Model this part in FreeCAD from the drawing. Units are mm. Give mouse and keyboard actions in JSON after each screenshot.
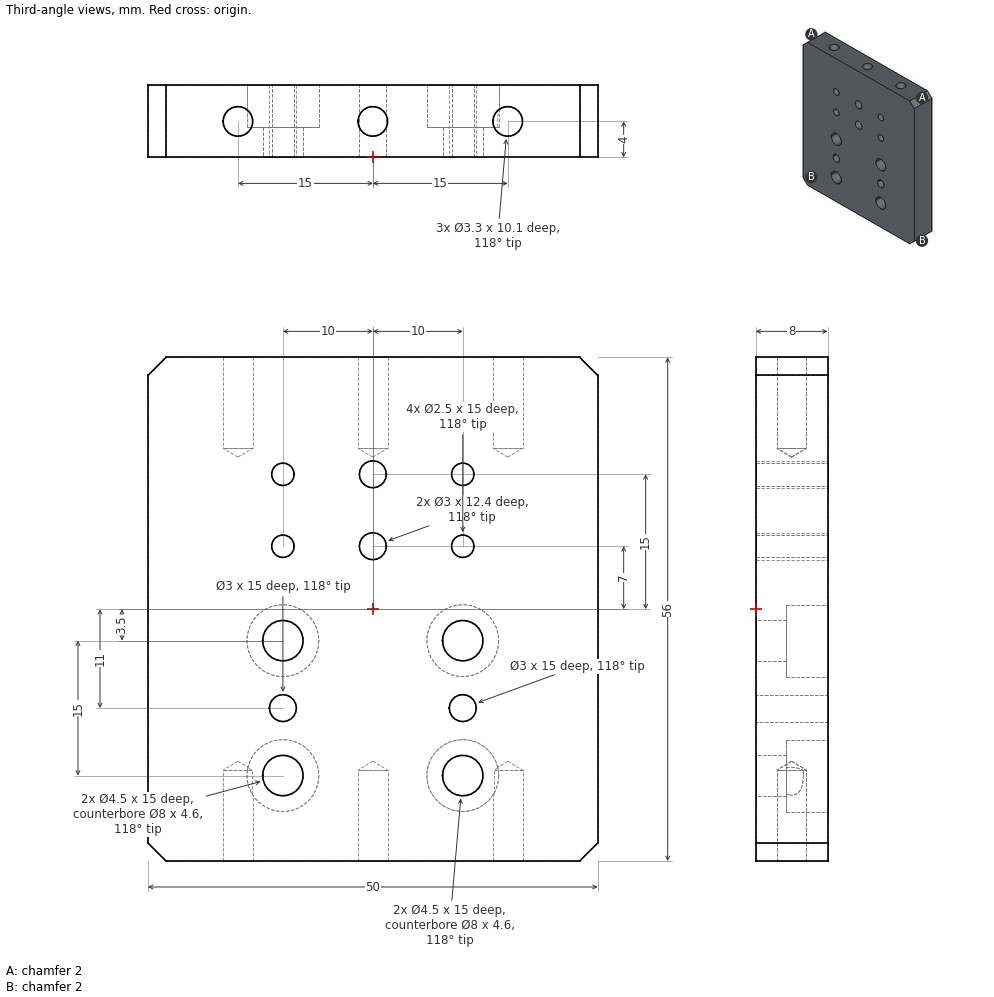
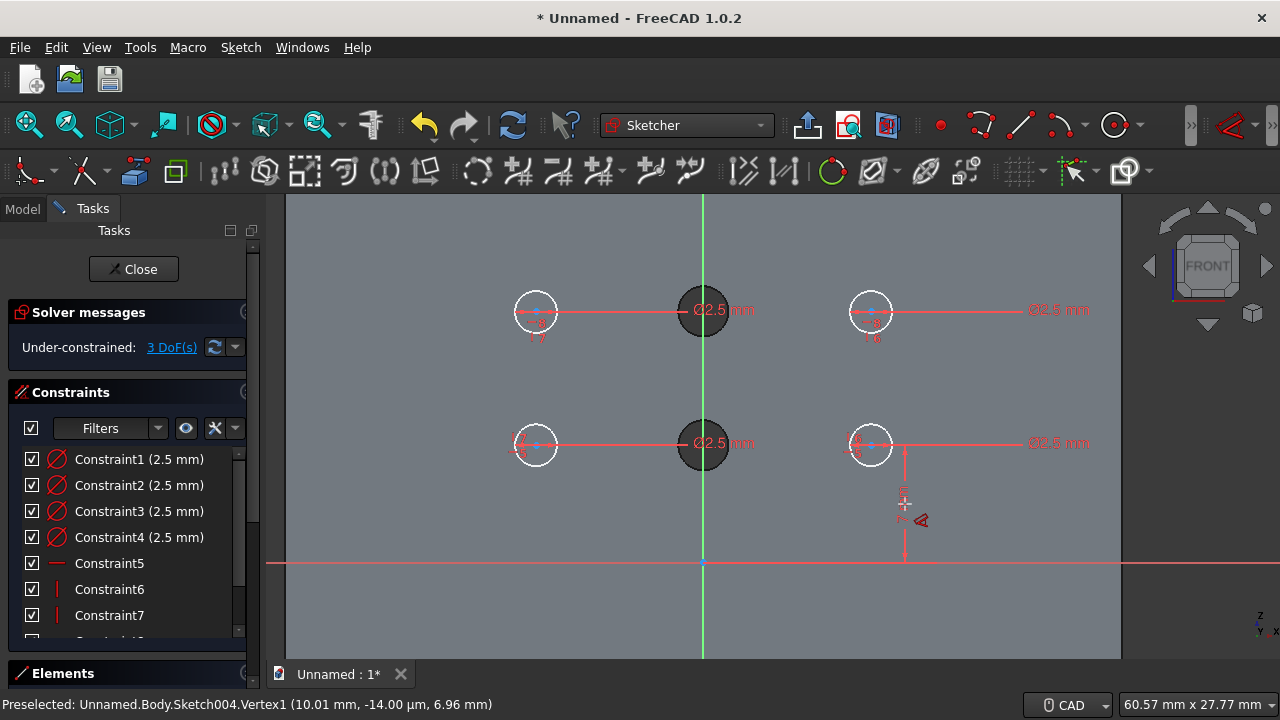
{"action": "left_click", "coordinate": [871, 445]}
{"action": "left_click", "coordinate": [787, 597]}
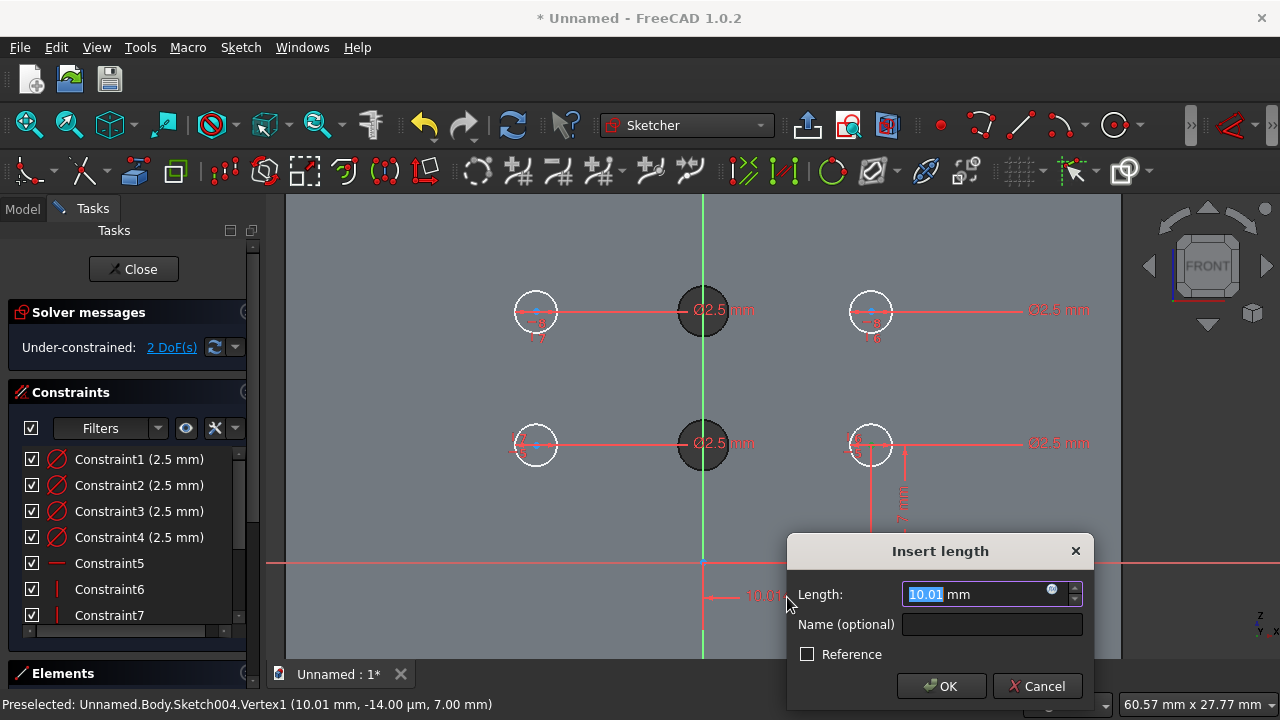
{"action": "type", "text": "10"}
{"action": "key", "text": "Return"}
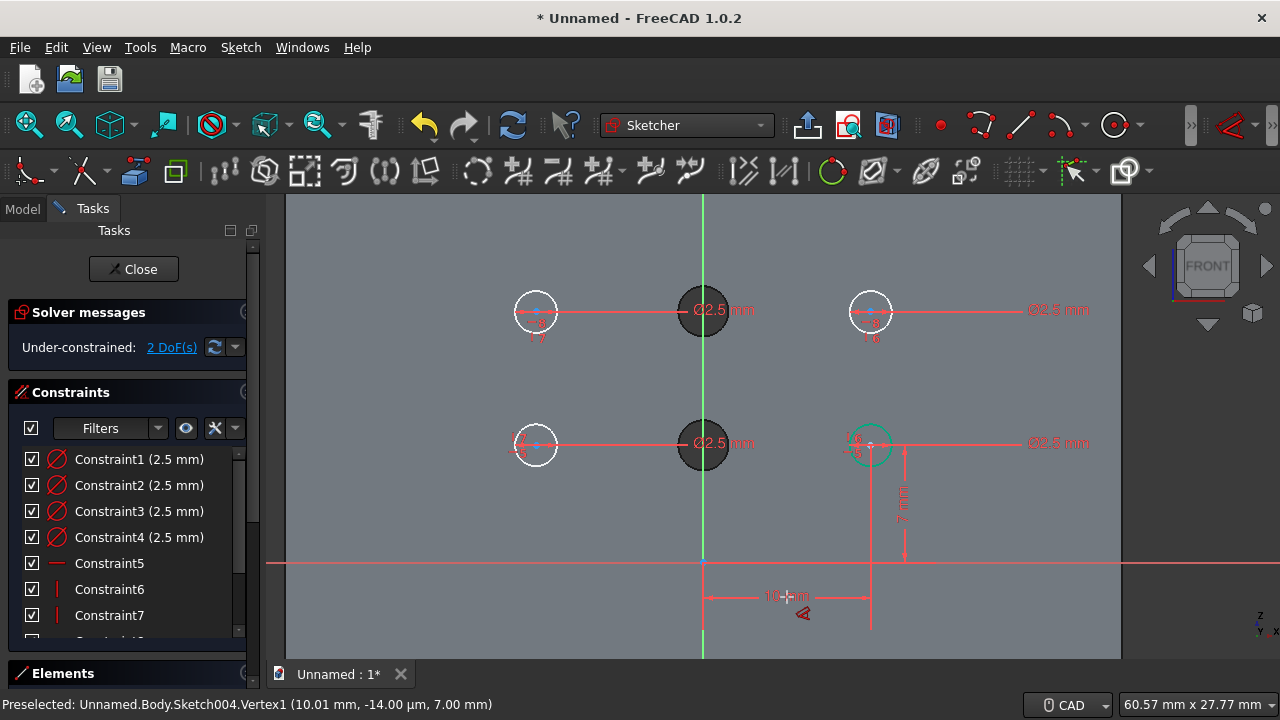
{"action": "left_click", "coordinate": [536, 445]}
{"action": "left_click", "coordinate": [620, 597]}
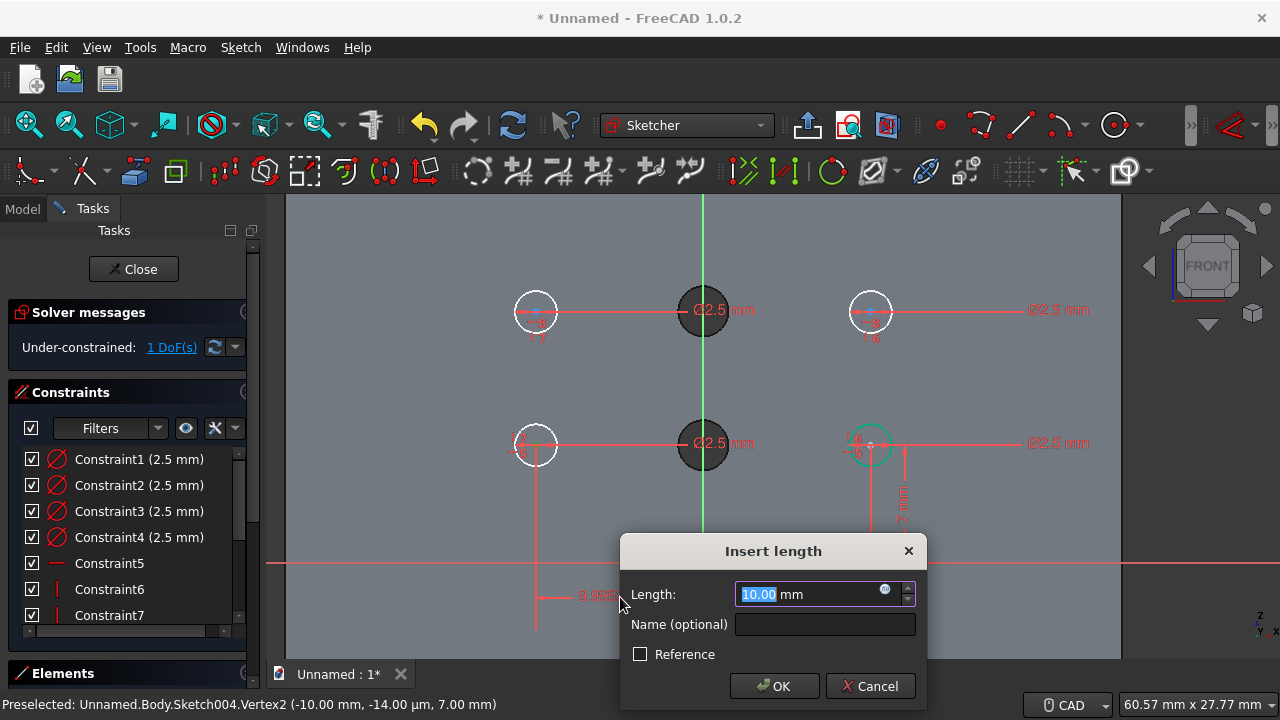
{"action": "type", "text": "10"}
{"action": "key", "text": "Return"}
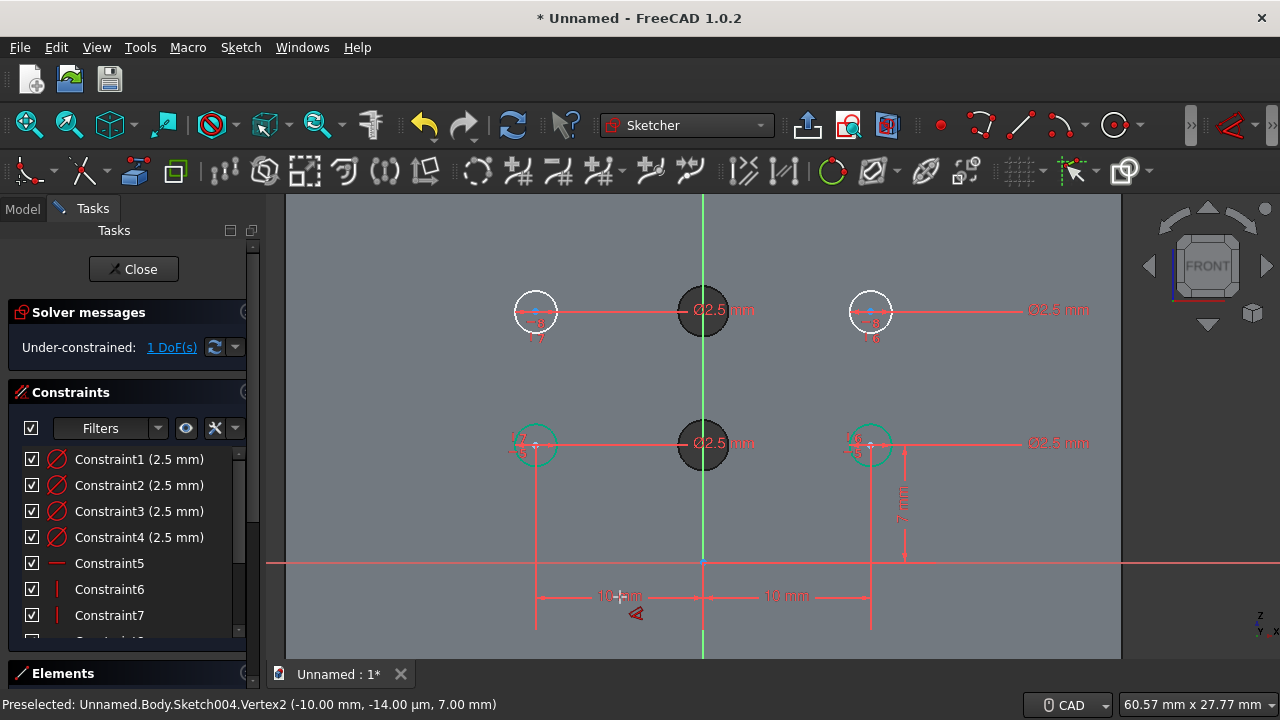
{"action": "left_click", "coordinate": [871, 312]}
{"action": "left_click", "coordinate": [905, 437]}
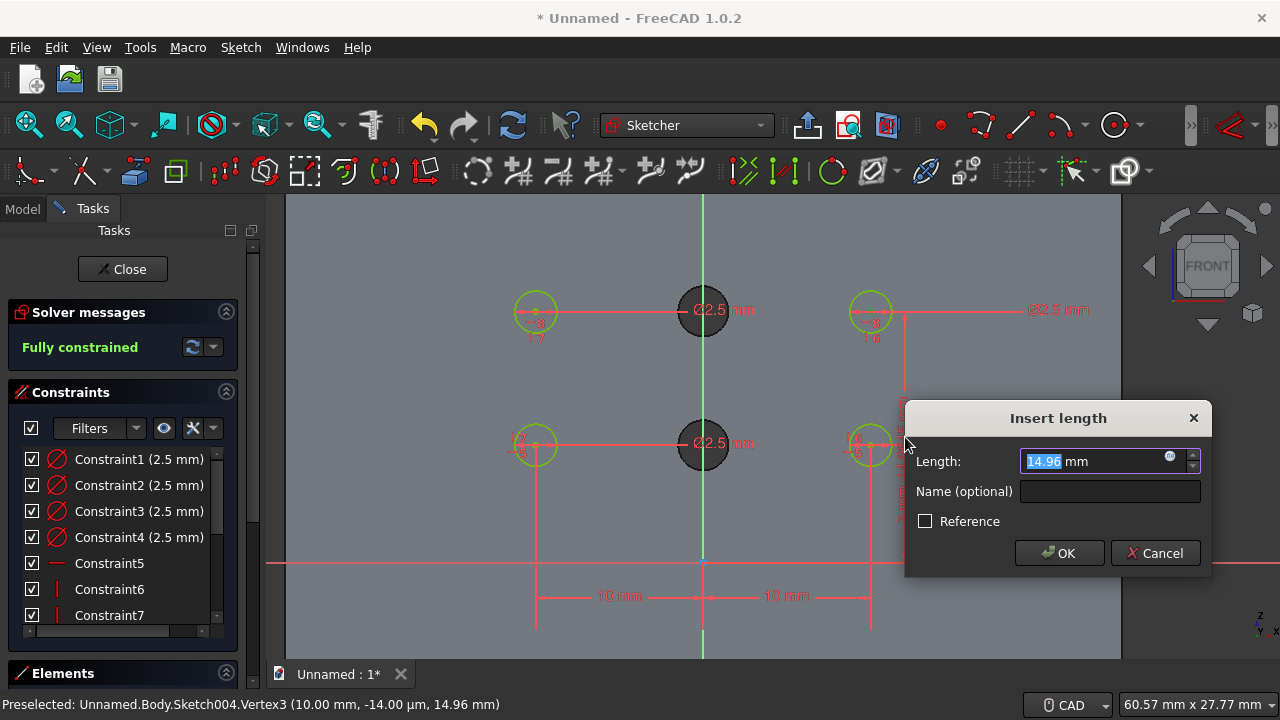
{"action": "type", "text": "15"}
{"action": "key", "text": "Return"}
{"action": "key", "text": "Escape"}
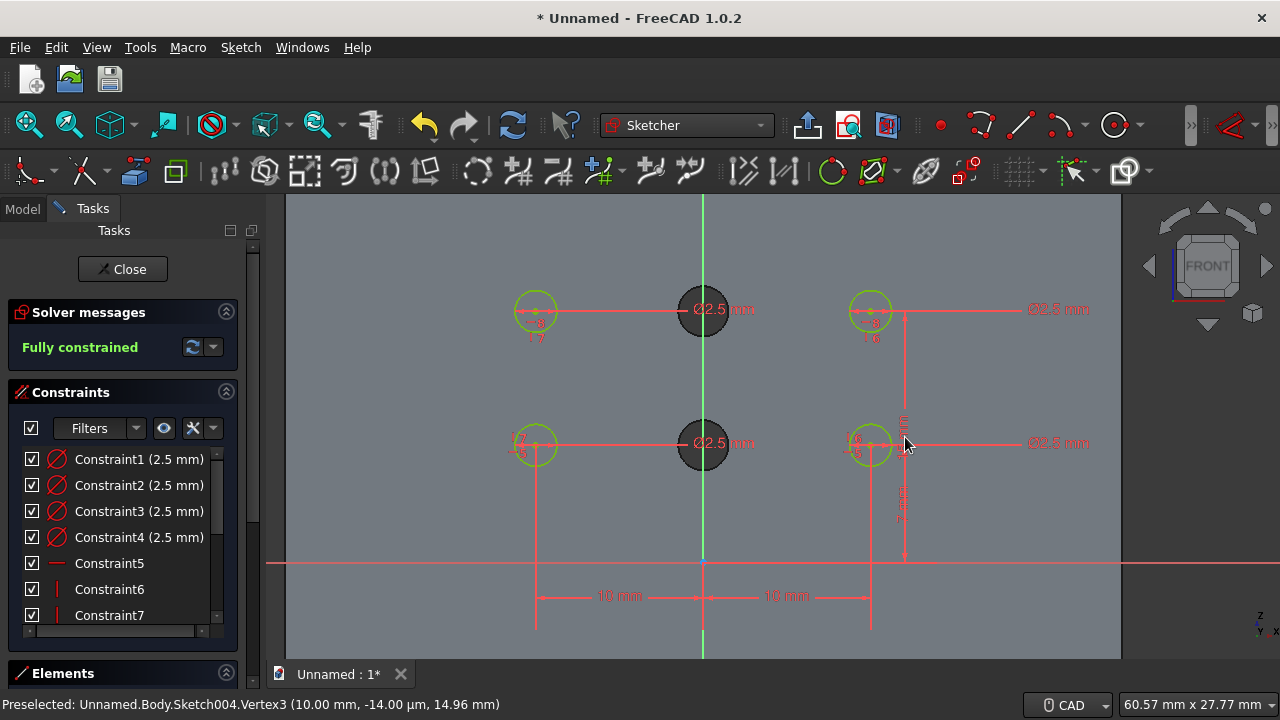
{"action": "left_click", "coordinate": [123, 269]}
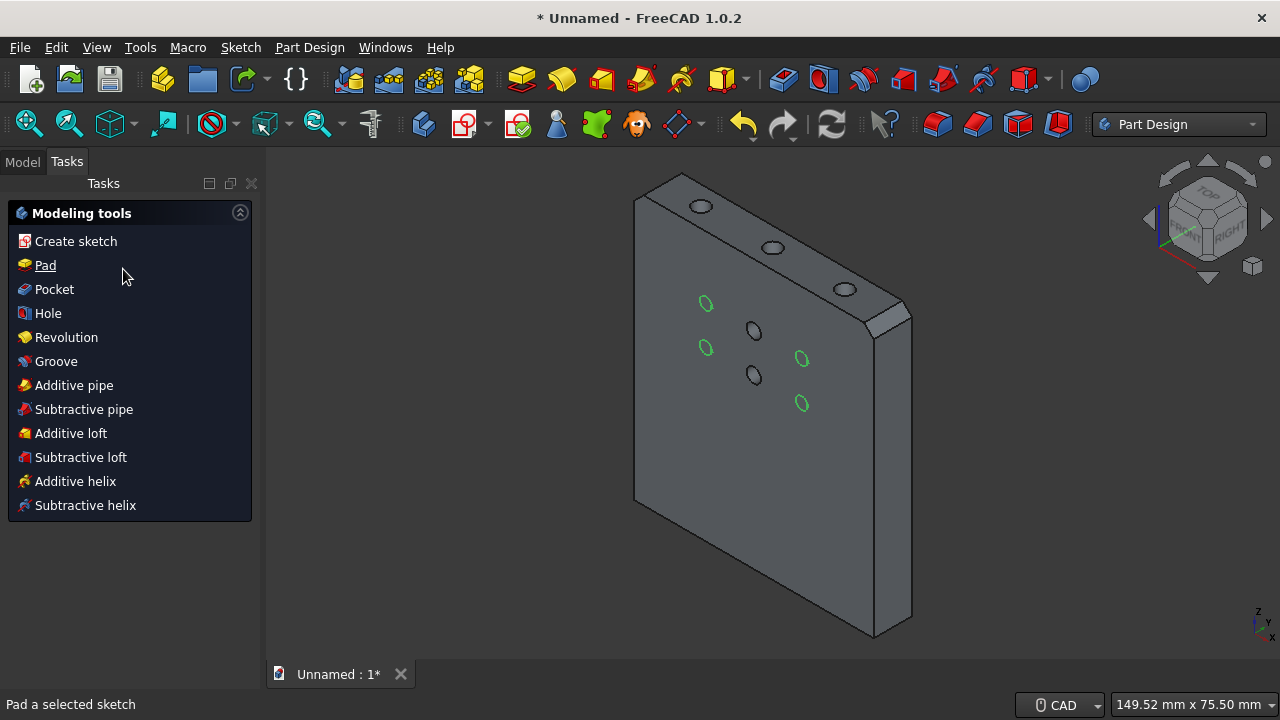
{"action": "left_click", "coordinate": [824, 80]}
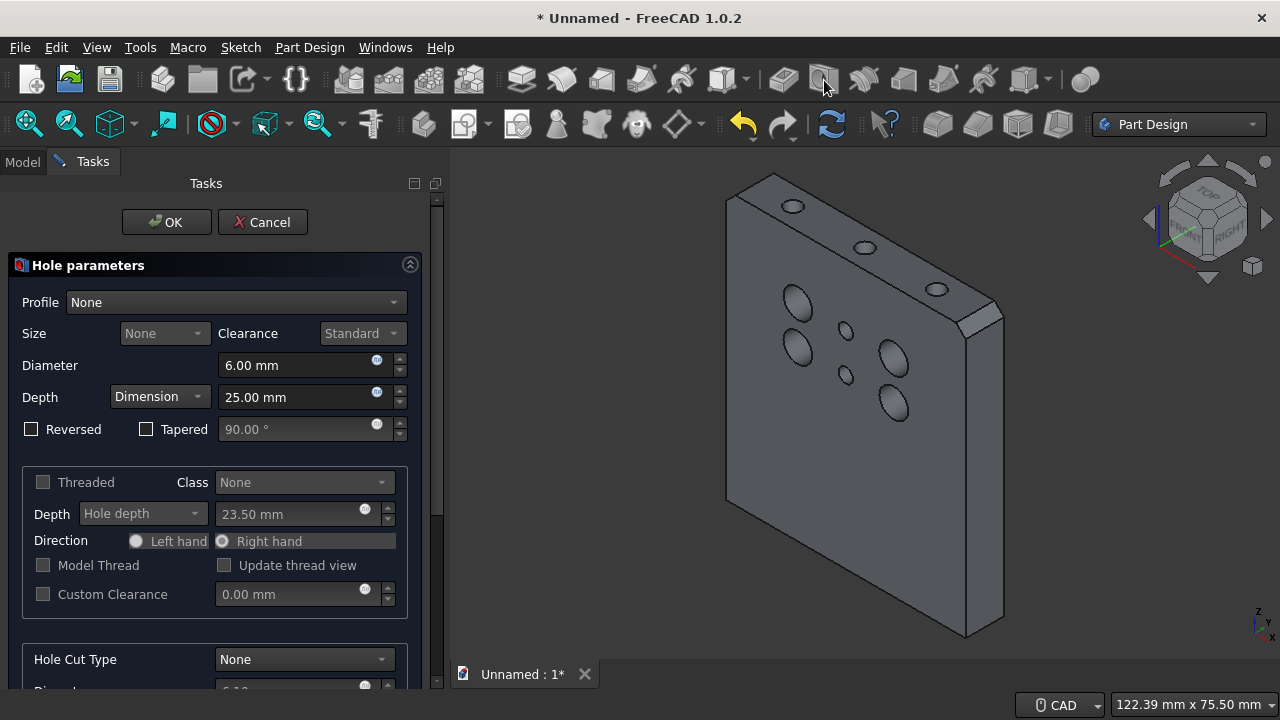
{"action": "triple_click", "coordinate": [305, 365]}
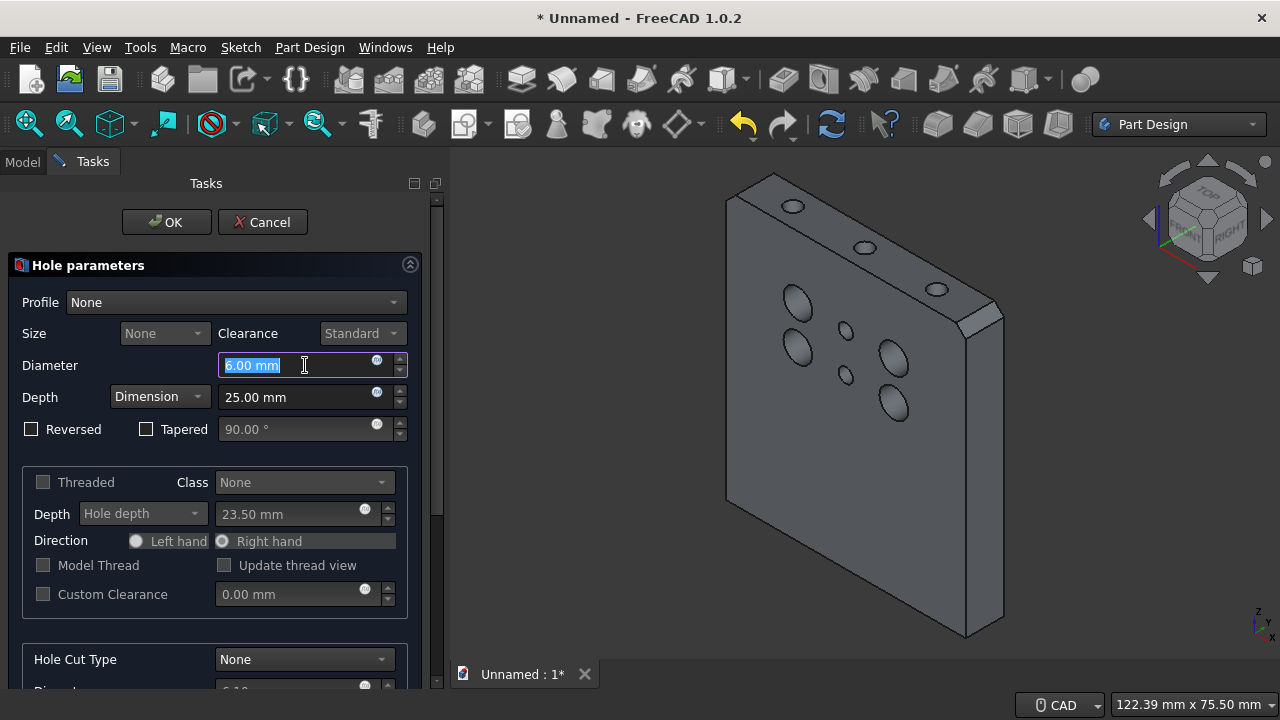
{"action": "type", "text": "2.5"}
{"action": "key", "text": "Tab"}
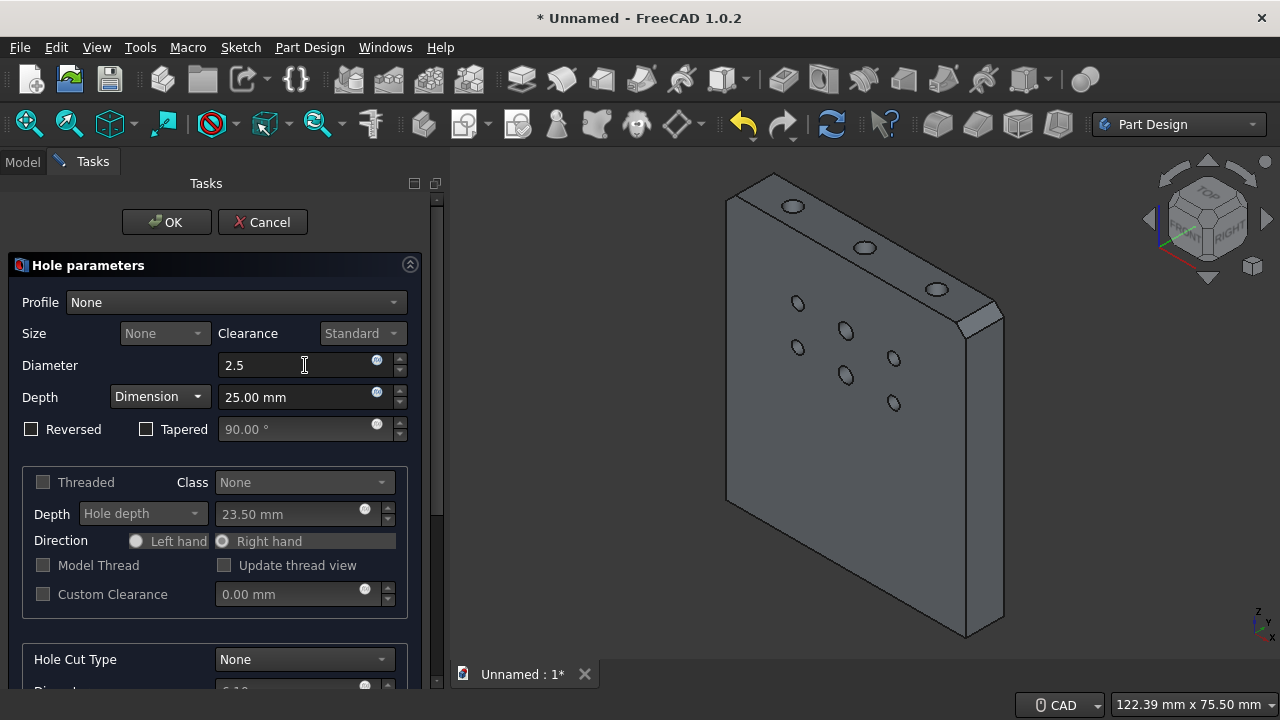
{"action": "triple_click", "coordinate": [305, 397]}